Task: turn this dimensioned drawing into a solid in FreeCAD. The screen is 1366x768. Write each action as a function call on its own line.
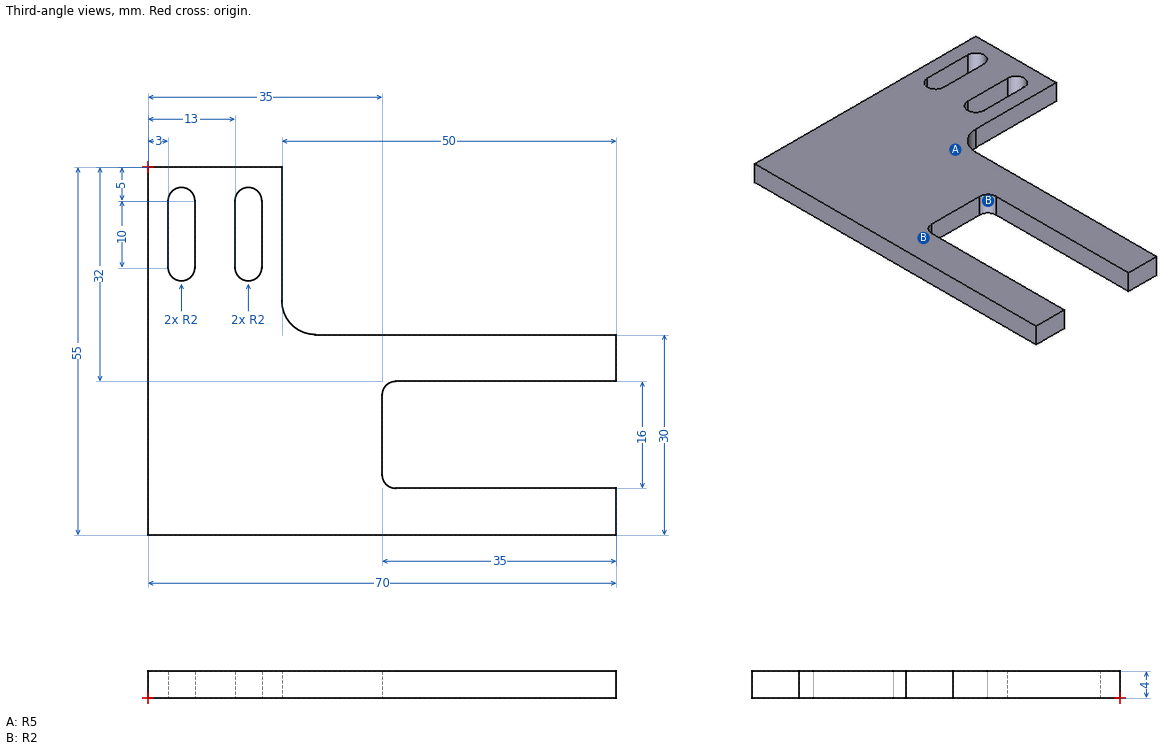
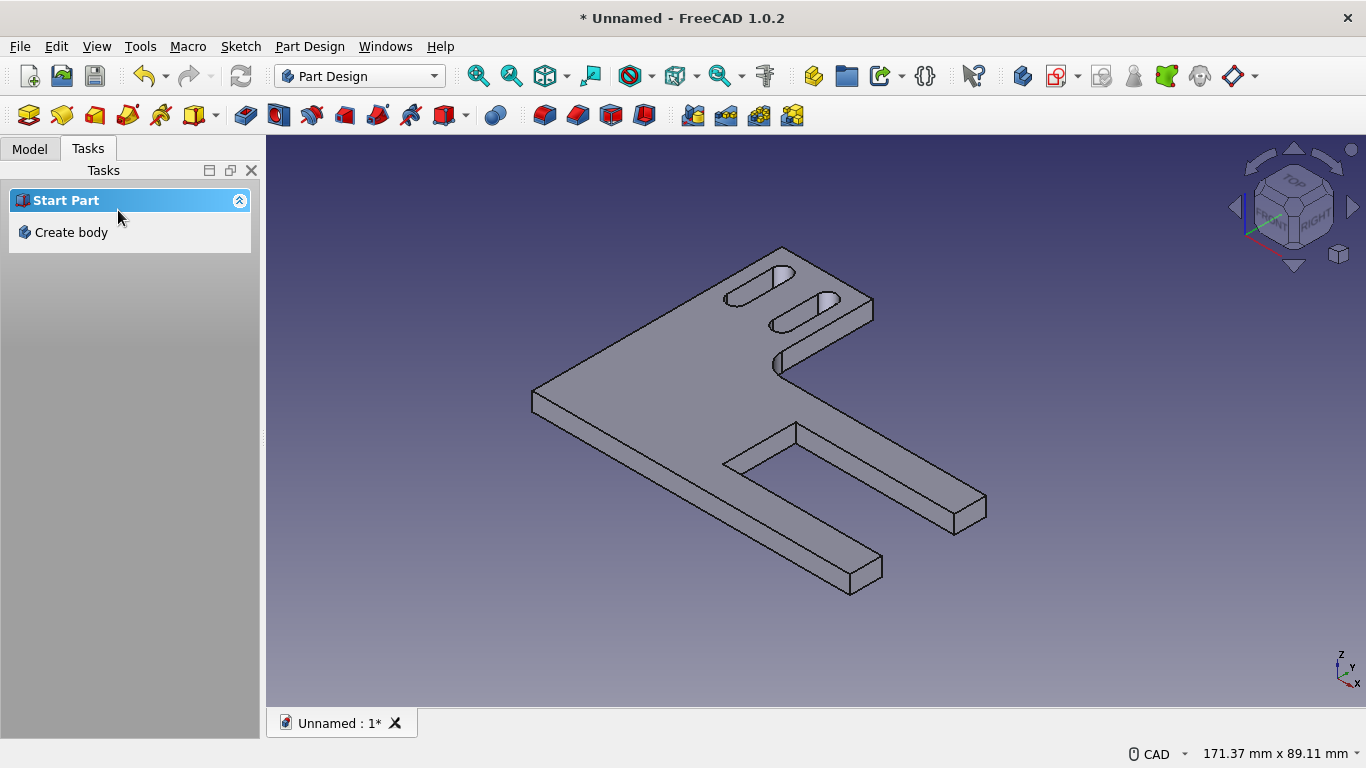
key(2)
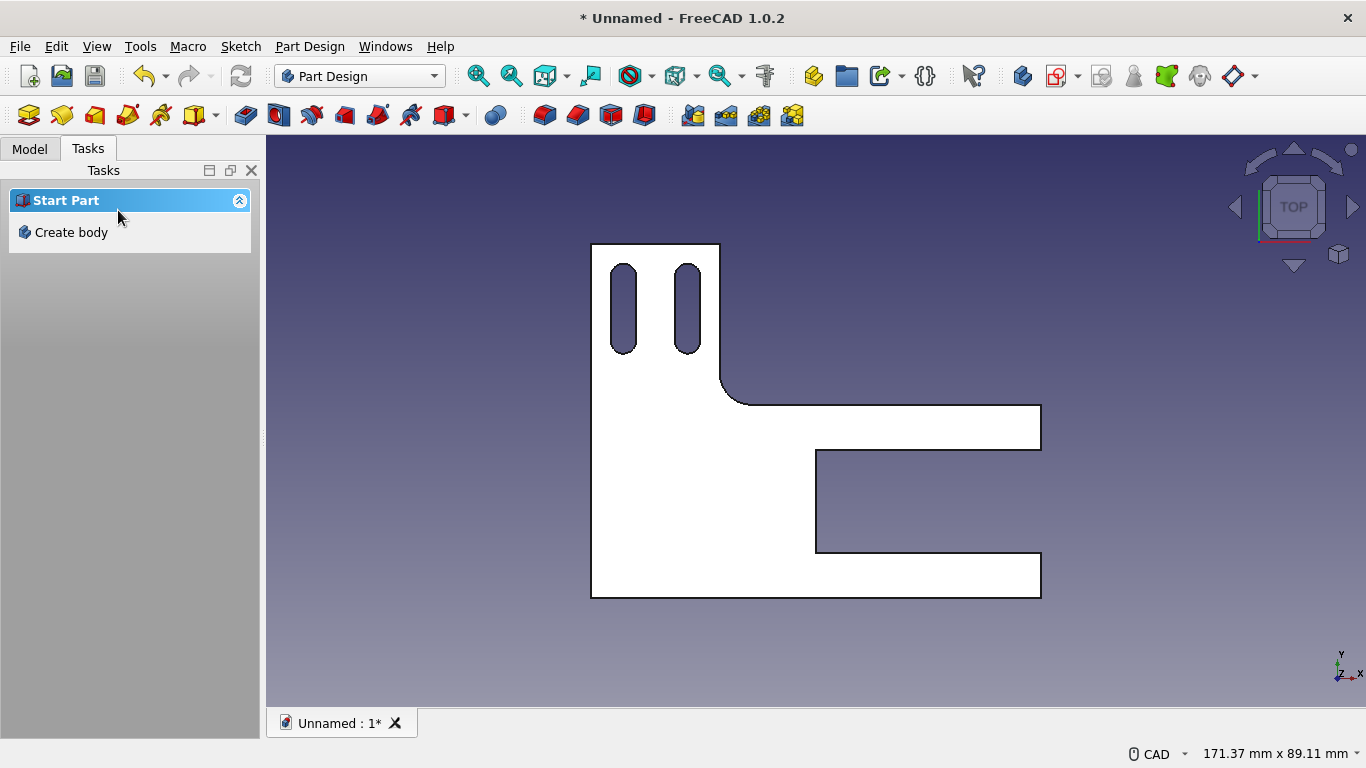
key(0)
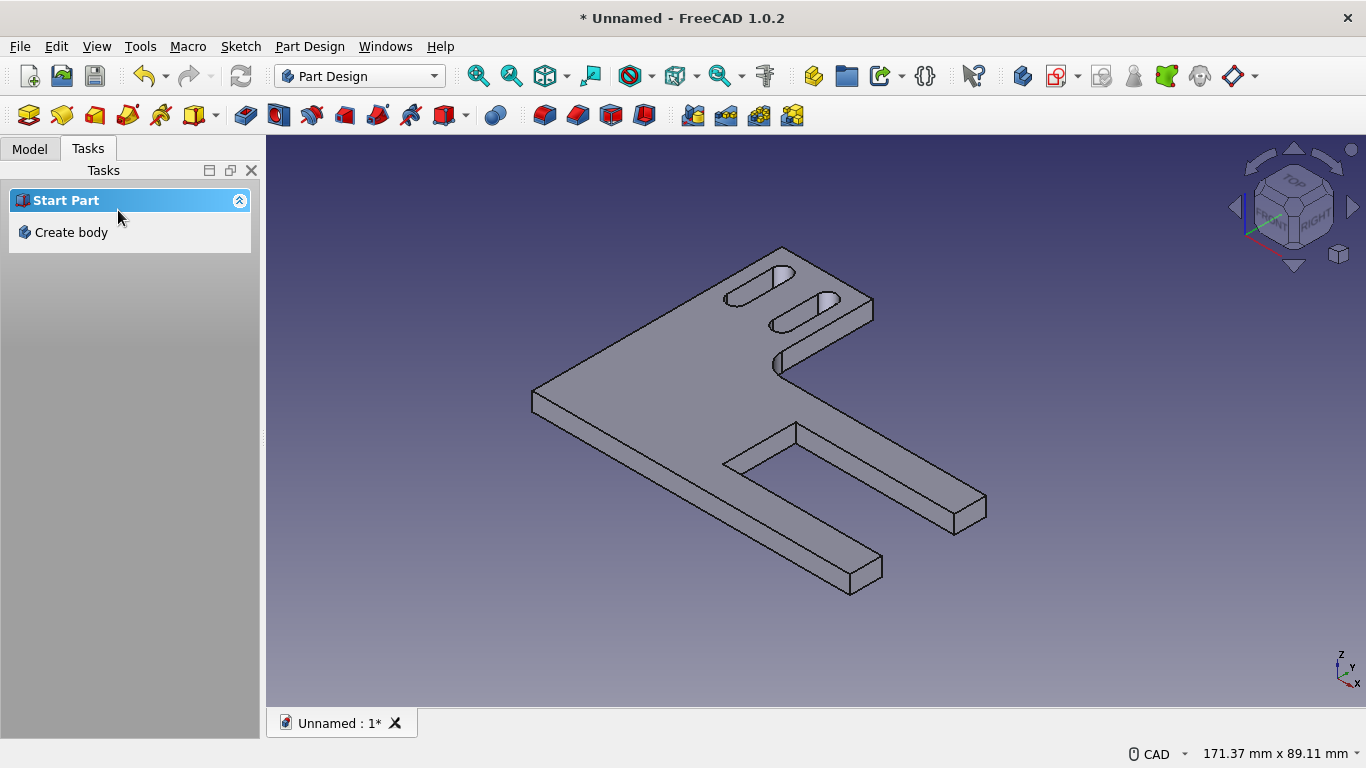
key(1)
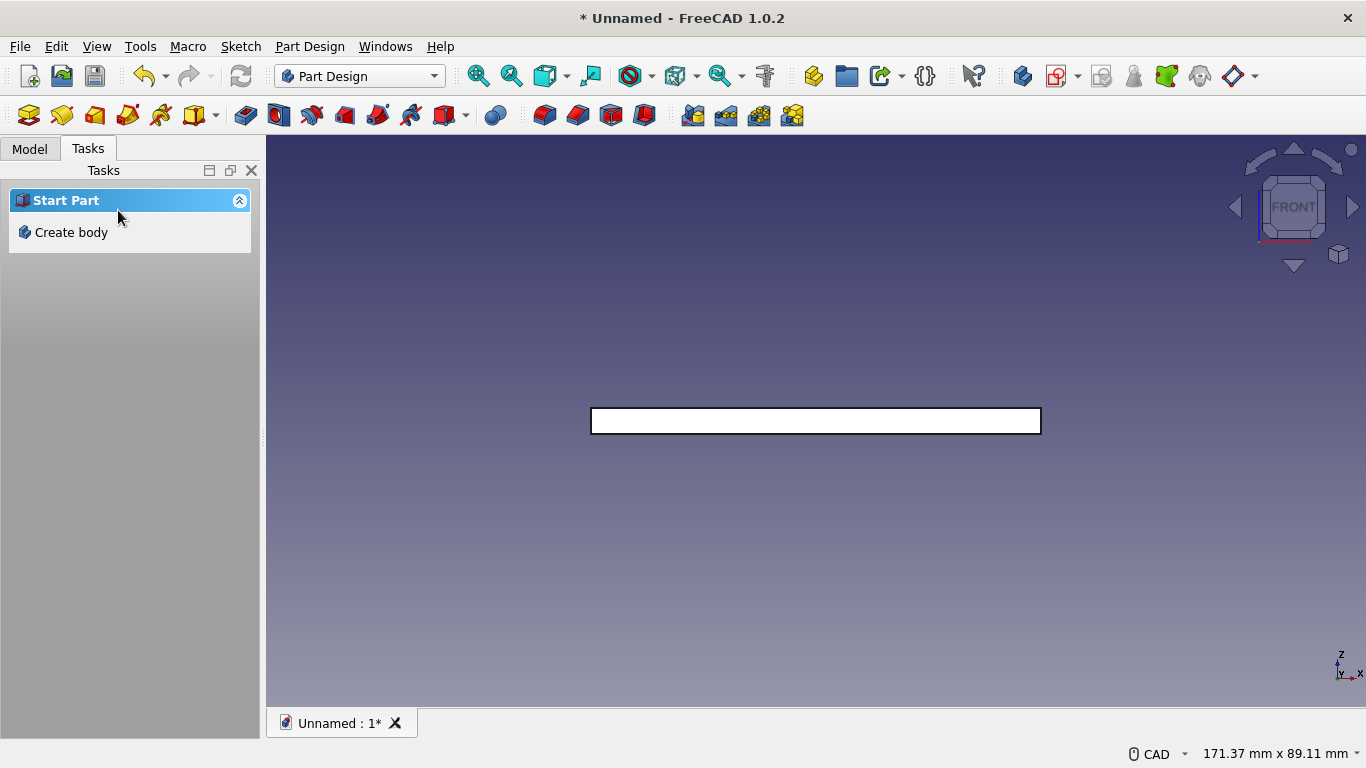
click(479, 76)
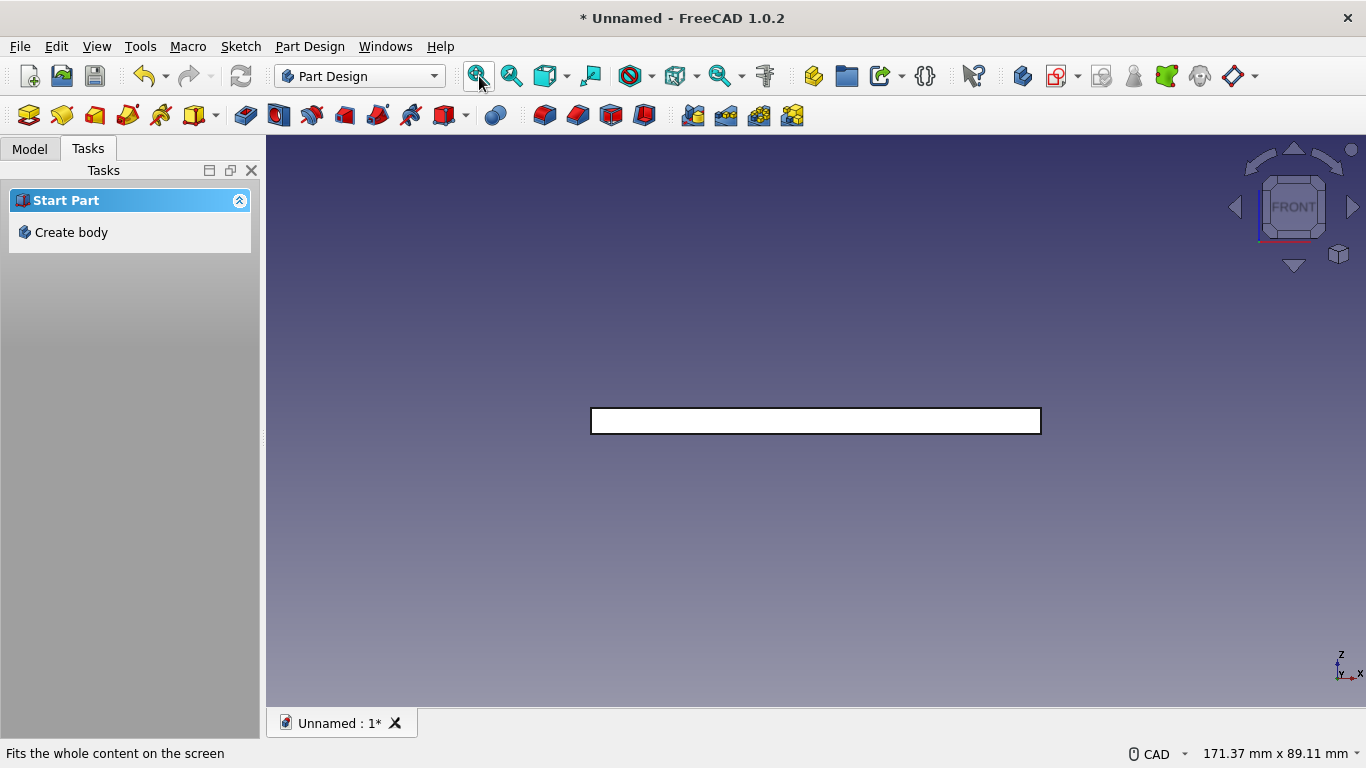
key(3)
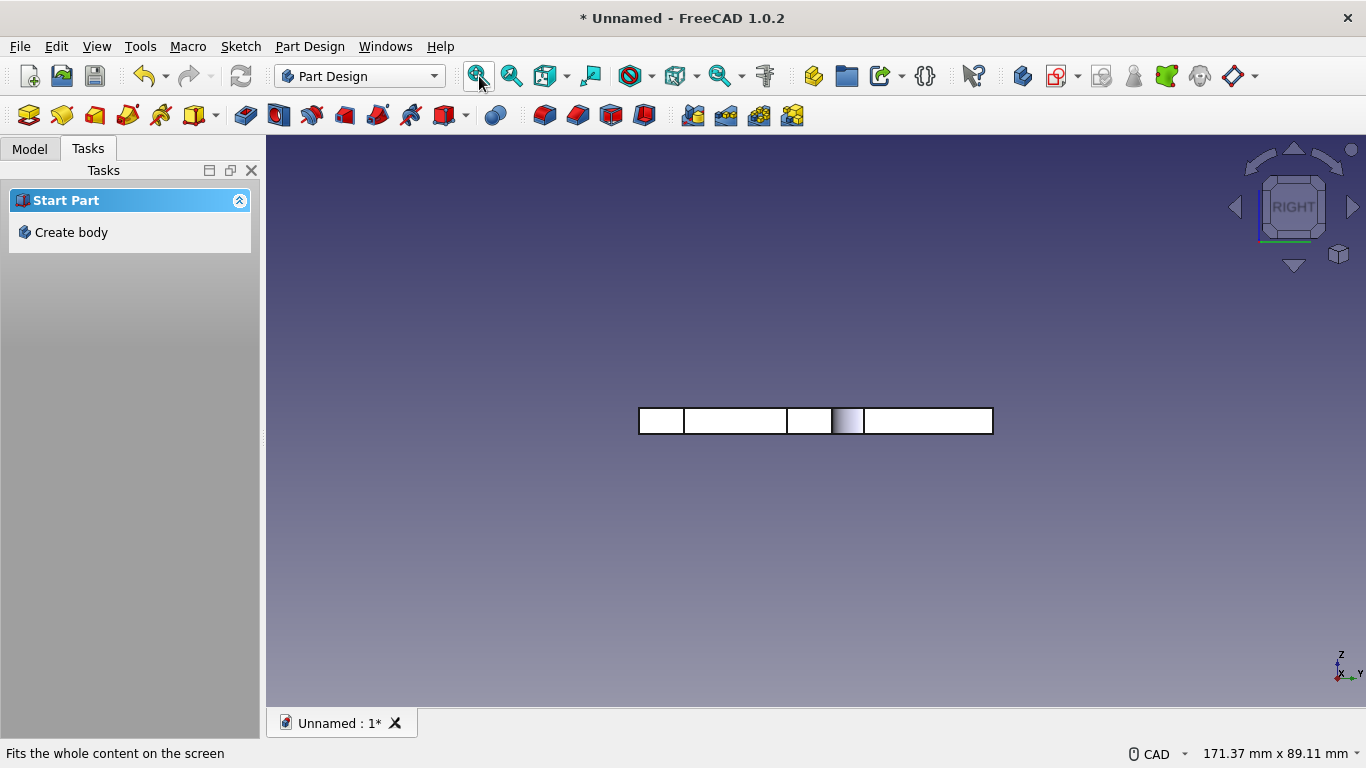
click(479, 76)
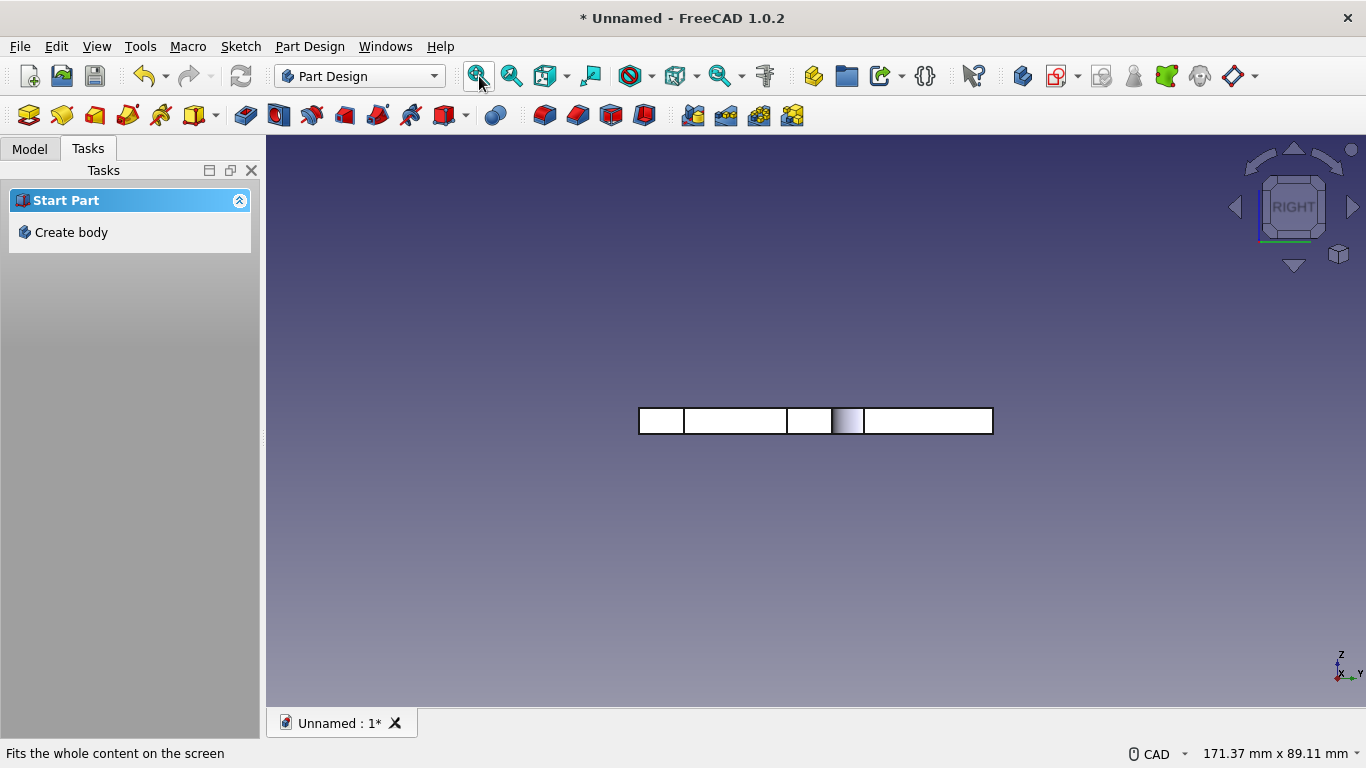
key(5)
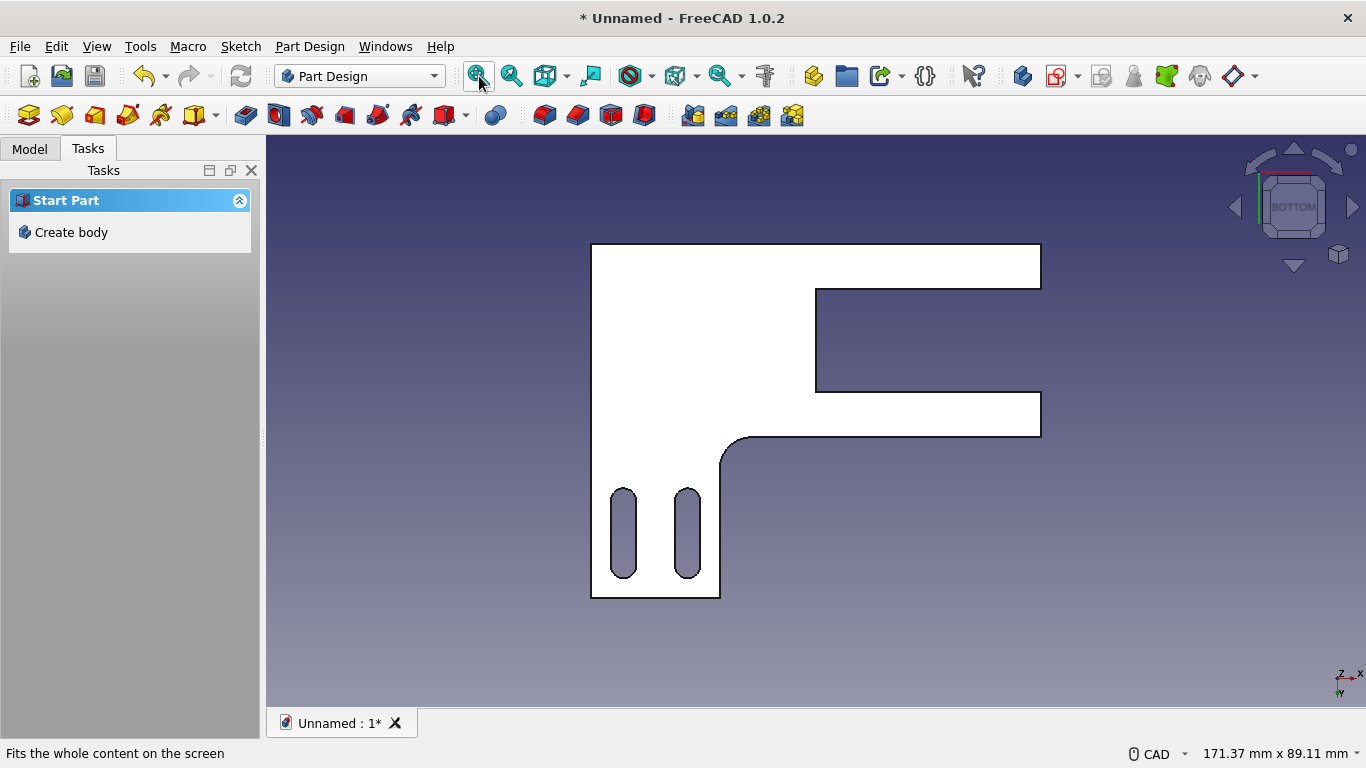
key(4)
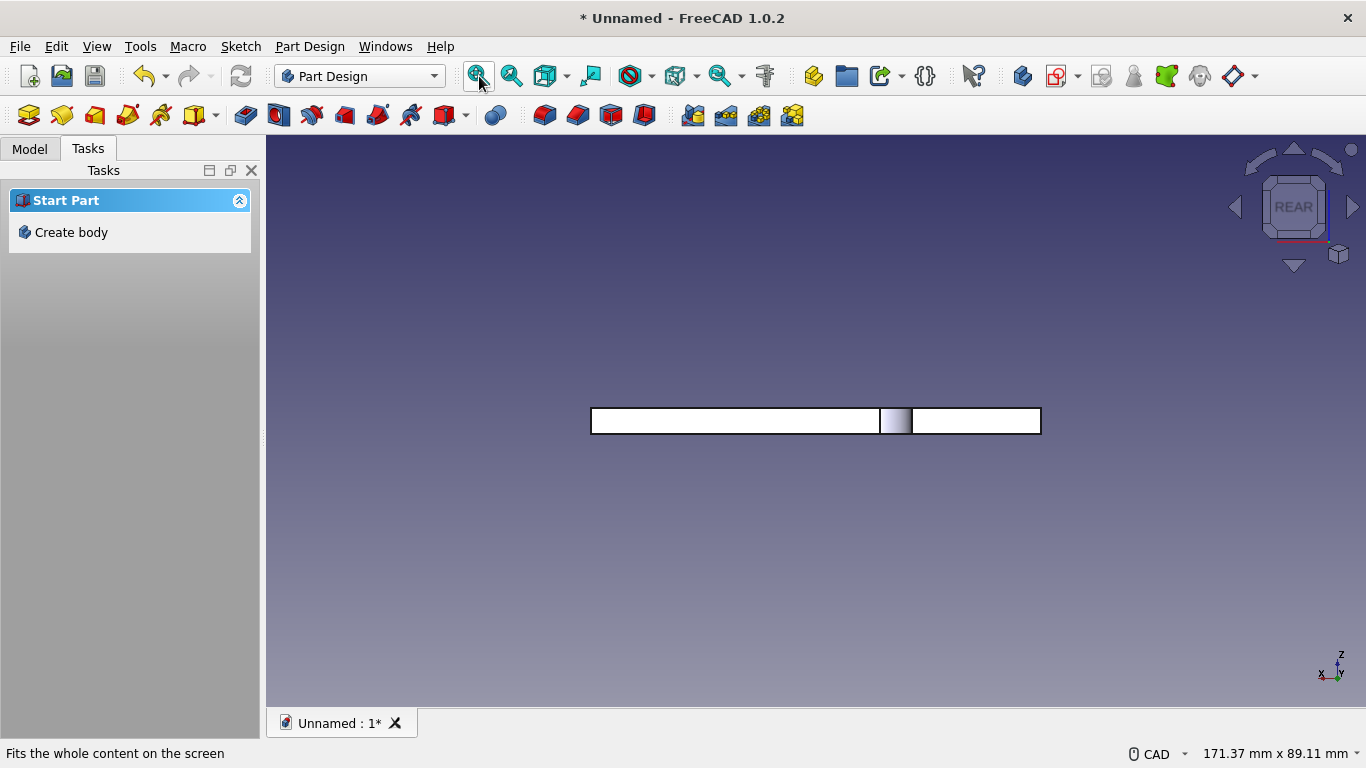
click(479, 76)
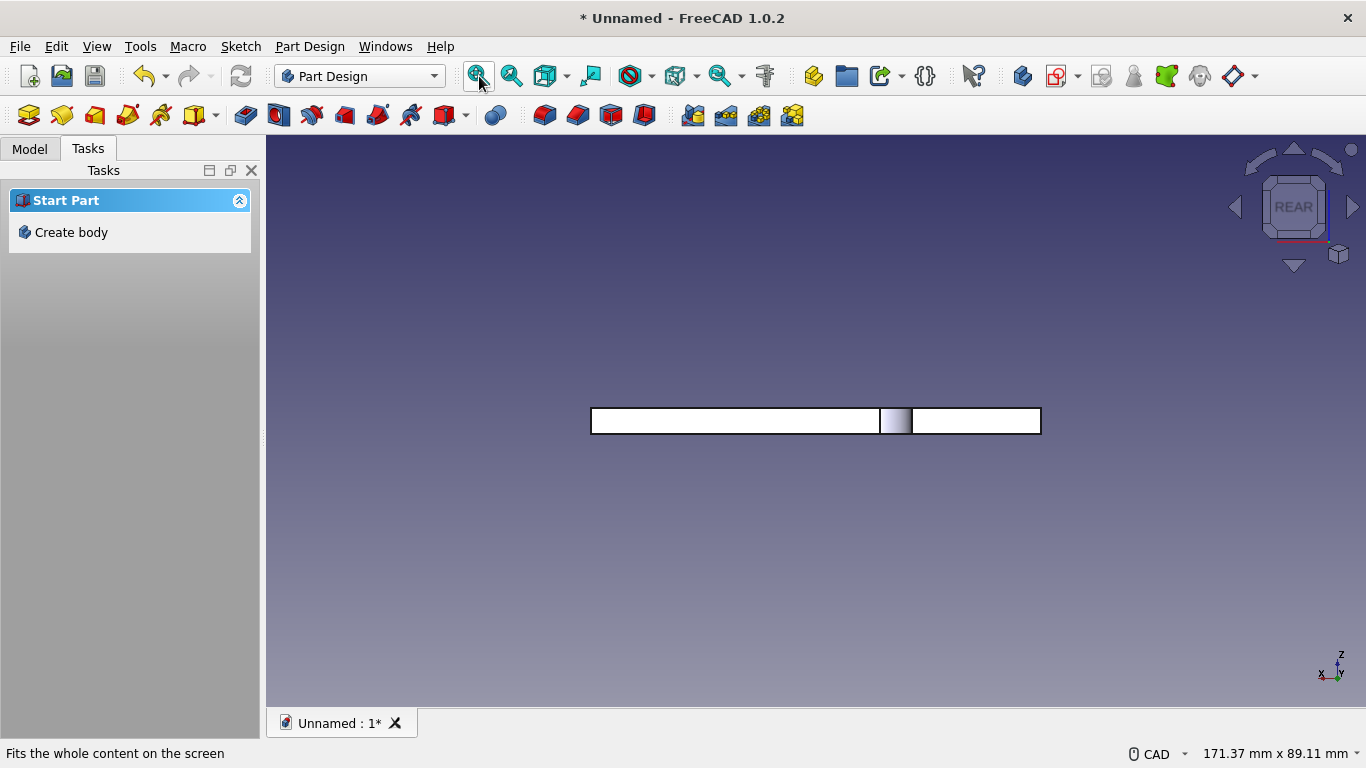
key(6)